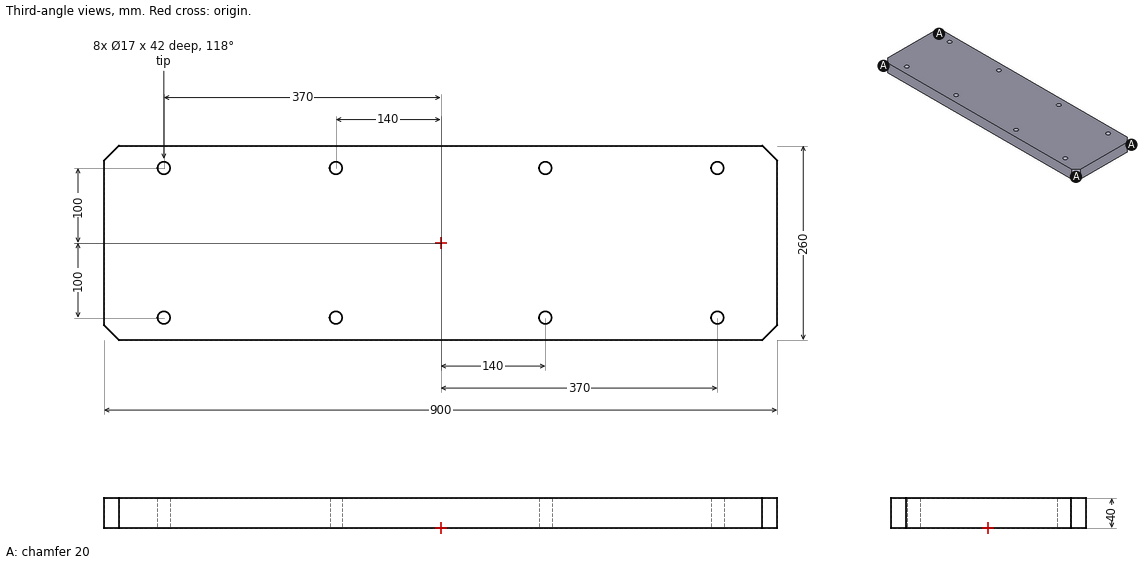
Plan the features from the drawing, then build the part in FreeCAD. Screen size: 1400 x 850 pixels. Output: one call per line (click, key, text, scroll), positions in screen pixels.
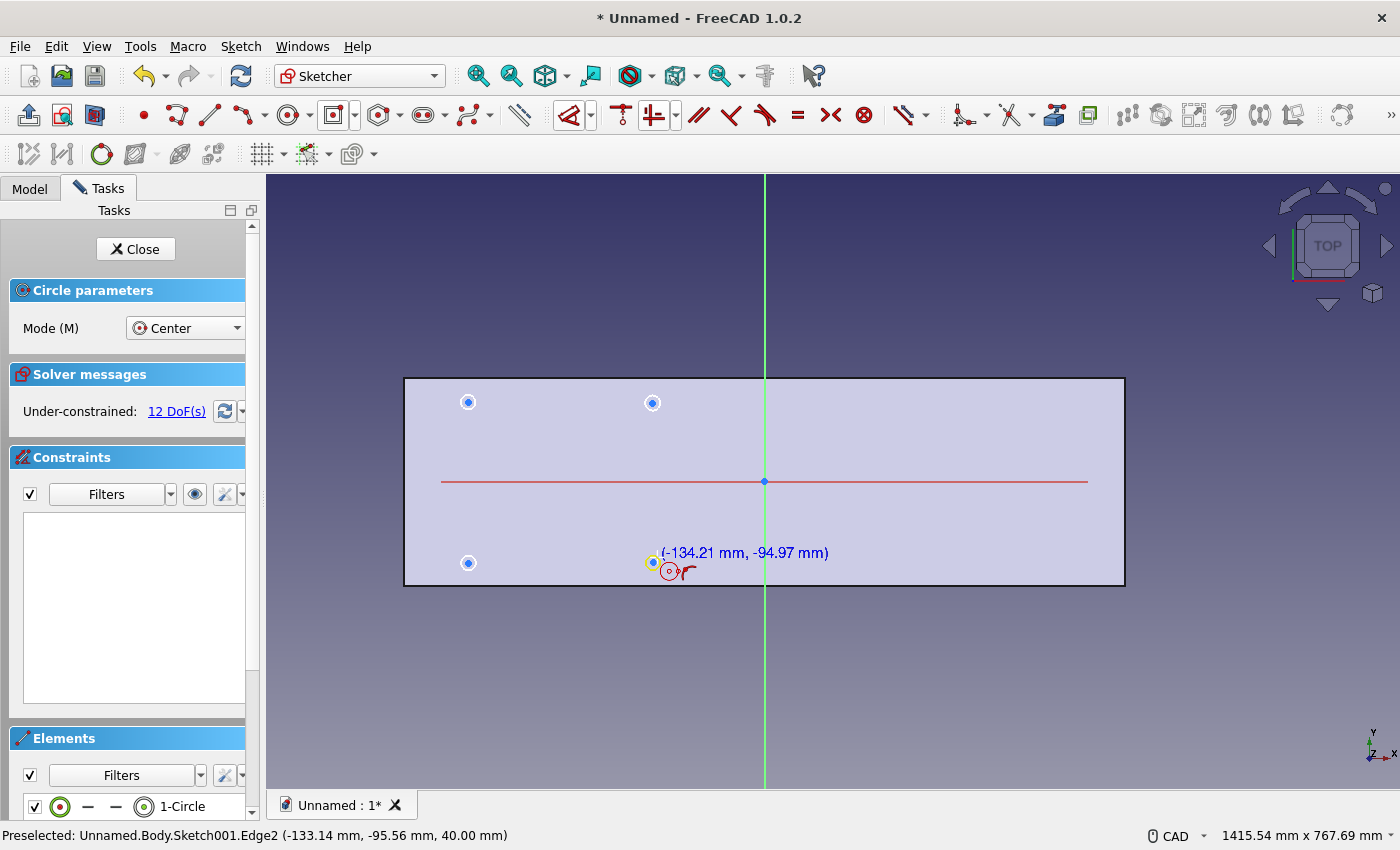
scroll(877, 562, up, 7)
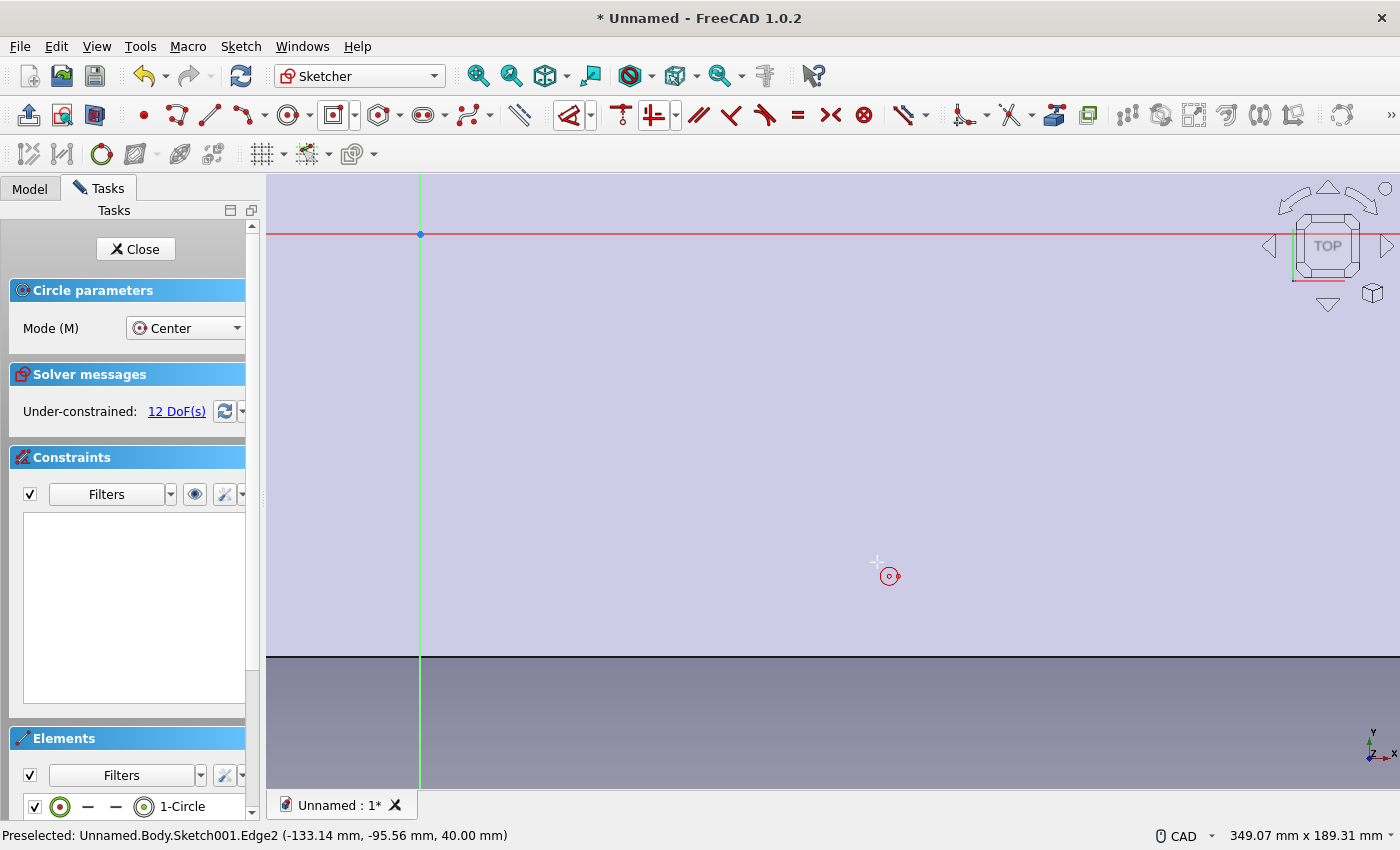
scroll(877, 562, down, 7)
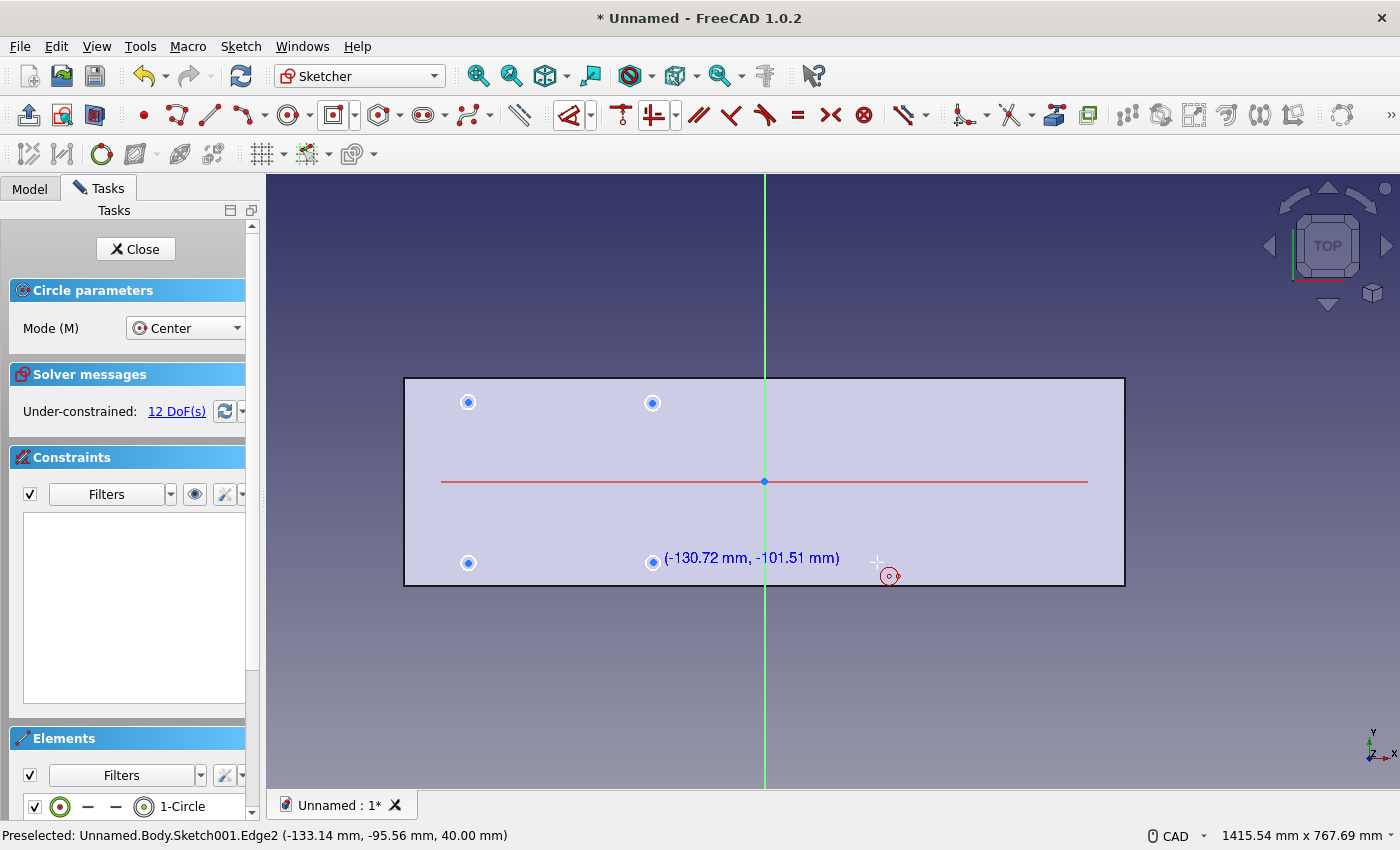
click(877, 562)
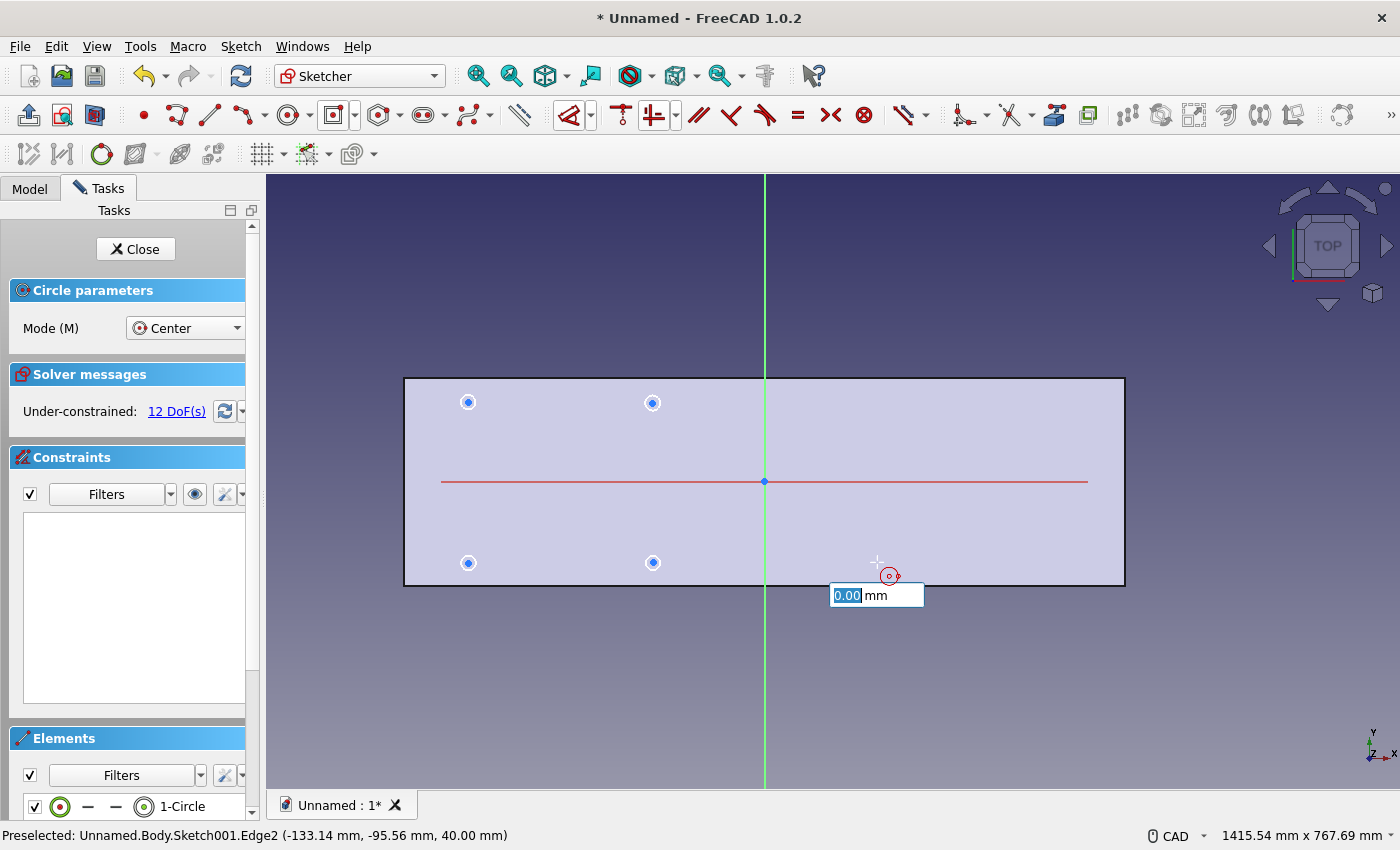
scroll(882, 557, up, 5)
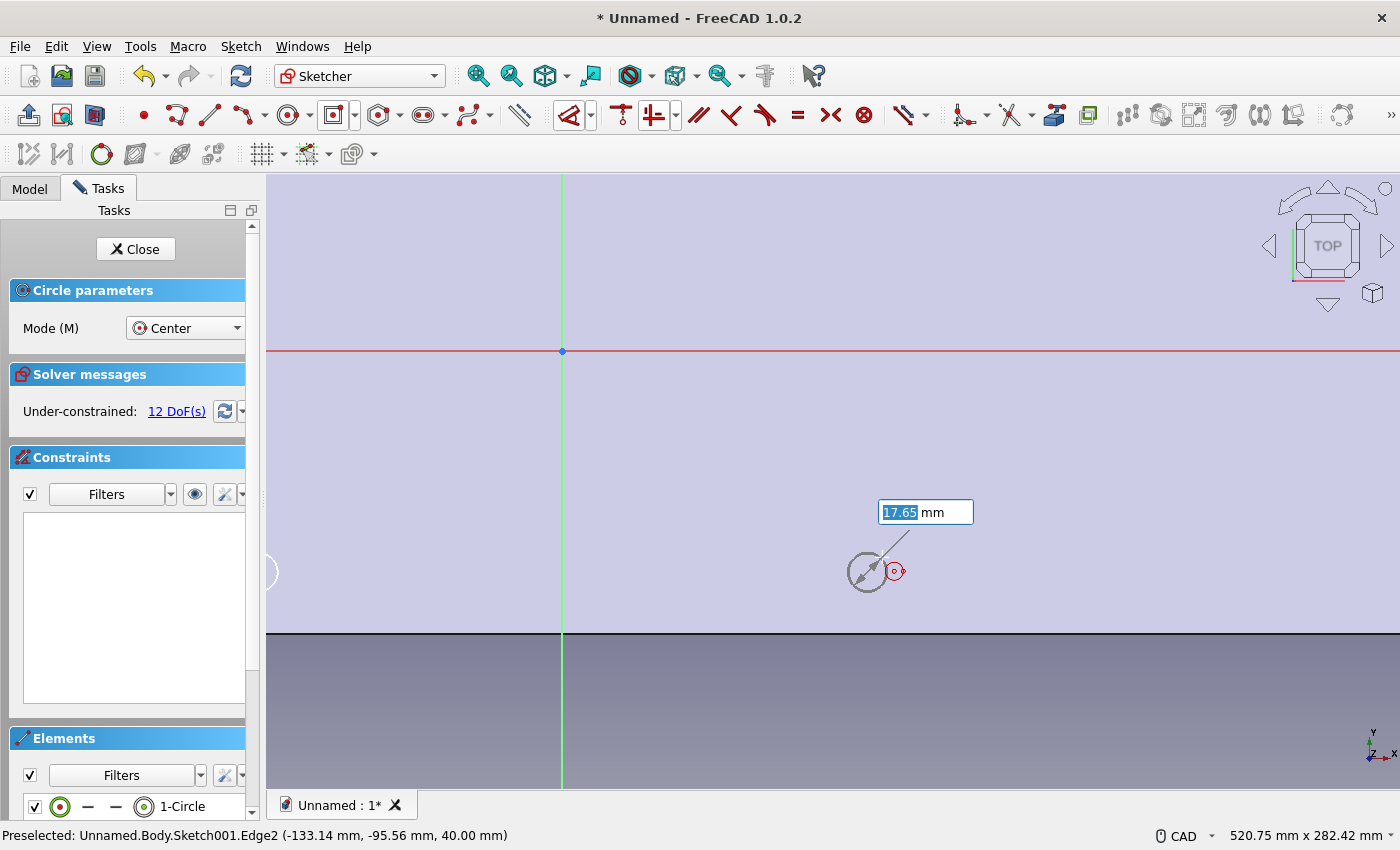
click(880, 556)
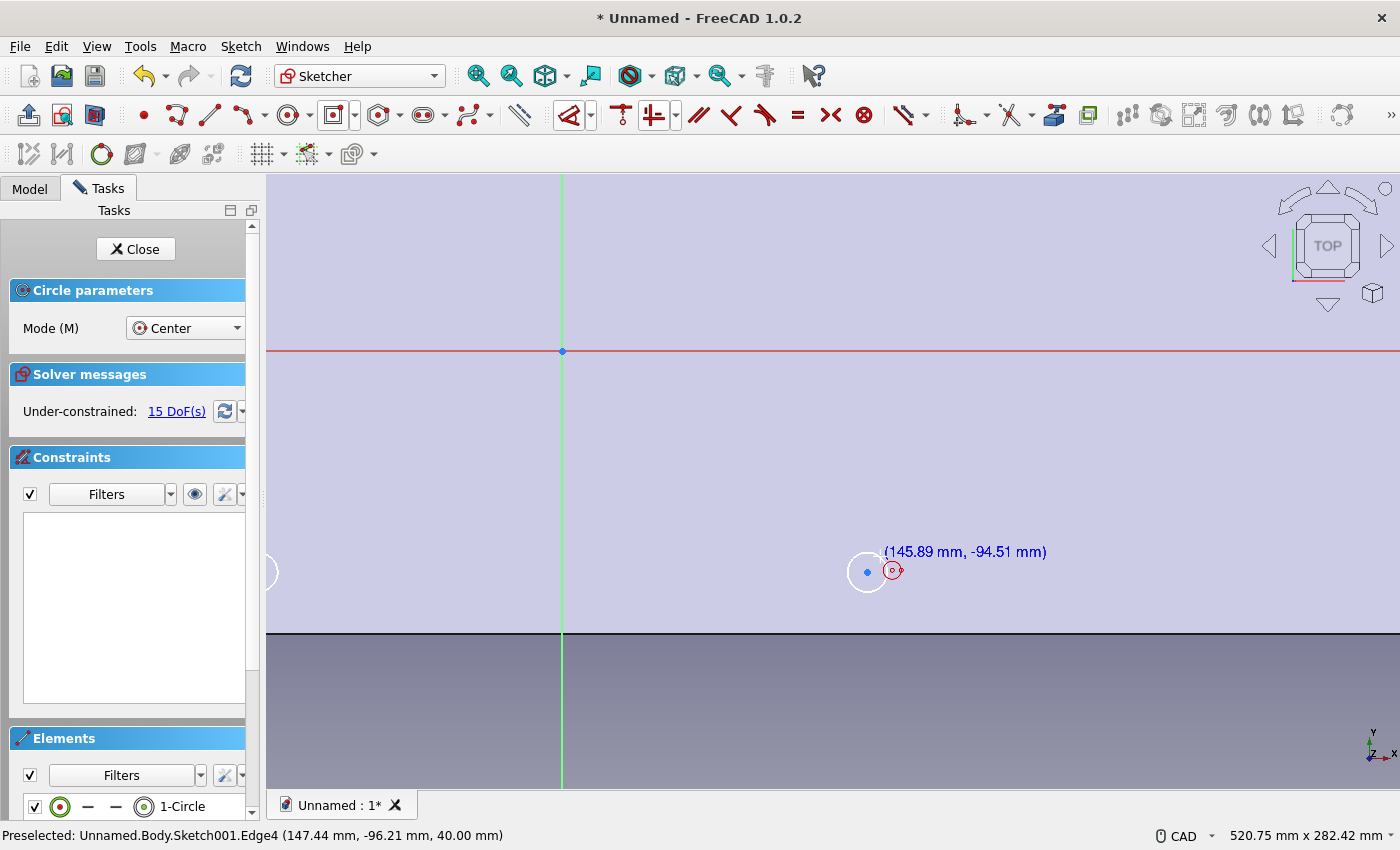
scroll(882, 557, down, 5)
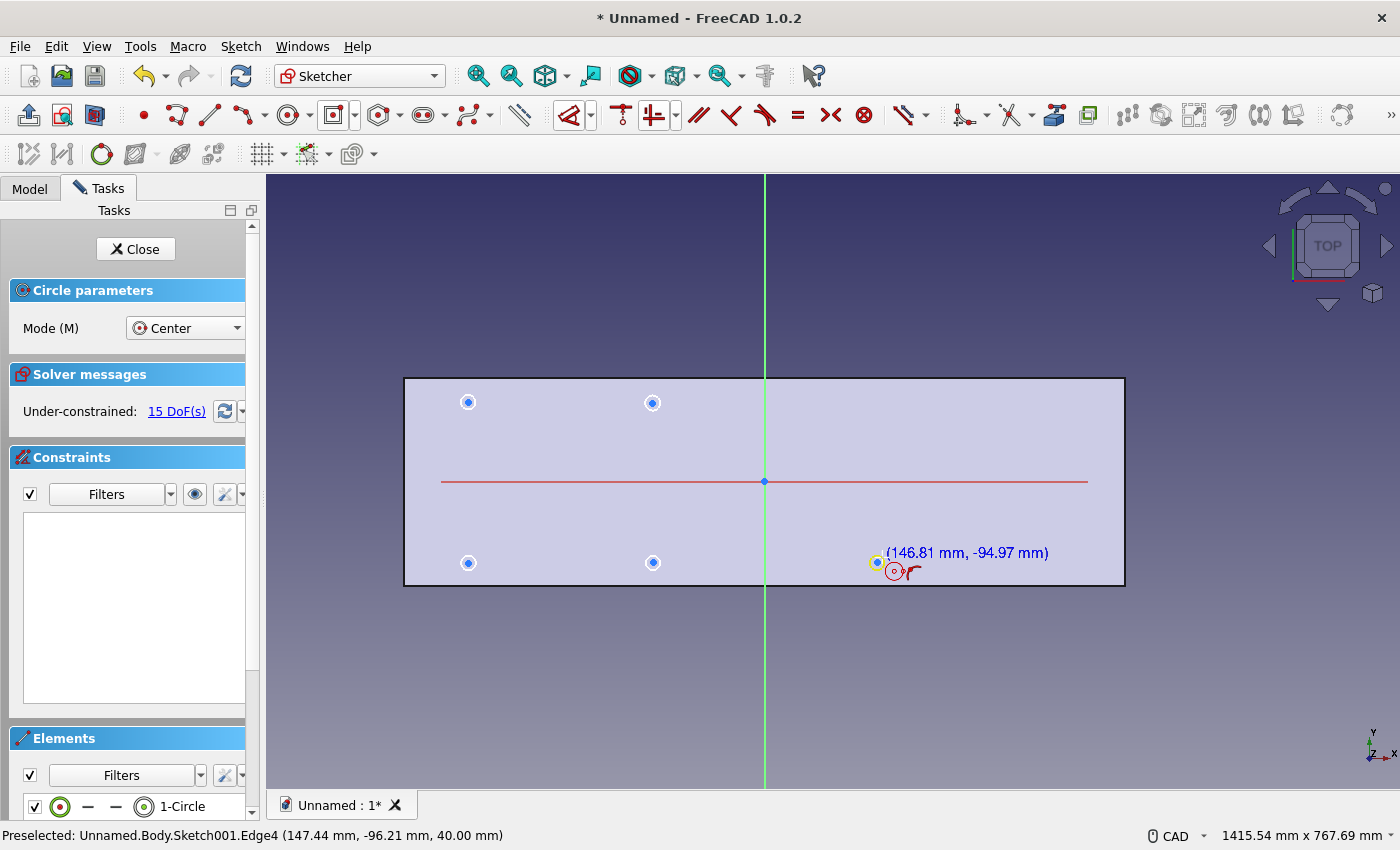
scroll(1061, 562, up, 7)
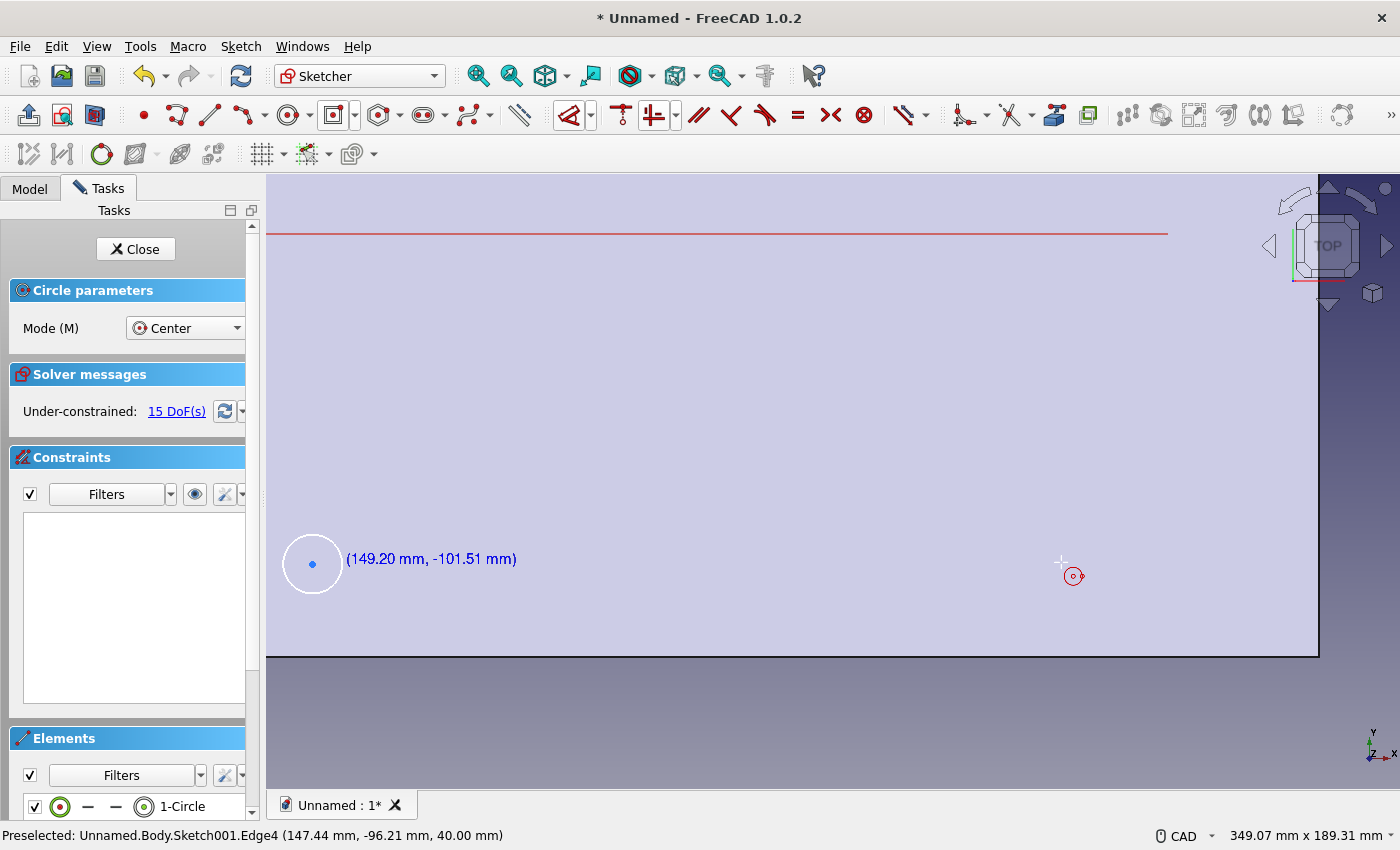
scroll(1061, 562, down, 7)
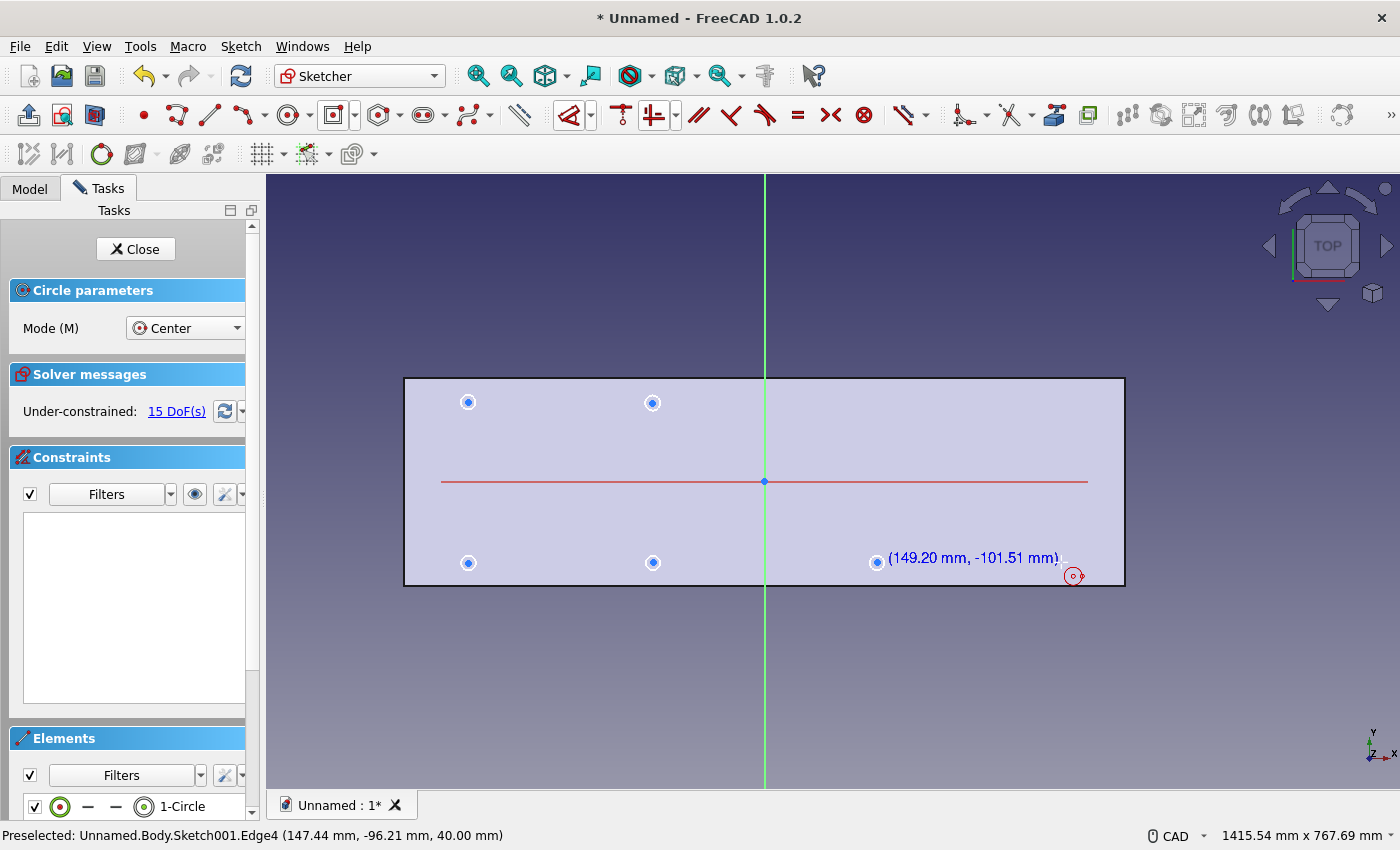
click(1061, 562)